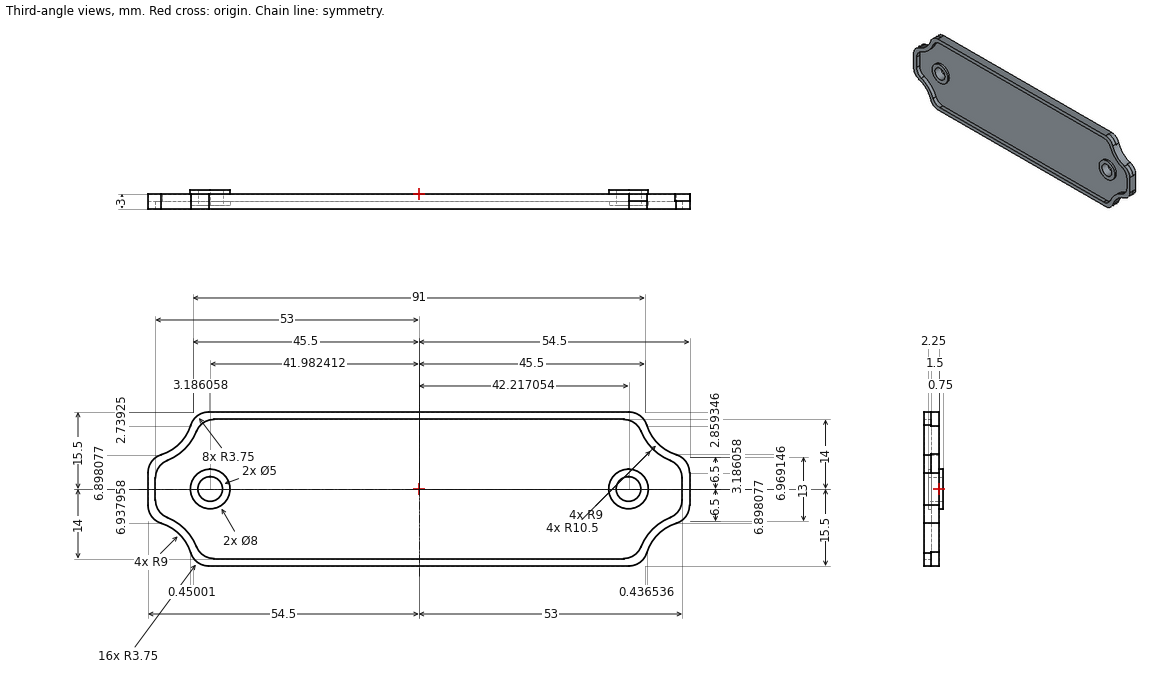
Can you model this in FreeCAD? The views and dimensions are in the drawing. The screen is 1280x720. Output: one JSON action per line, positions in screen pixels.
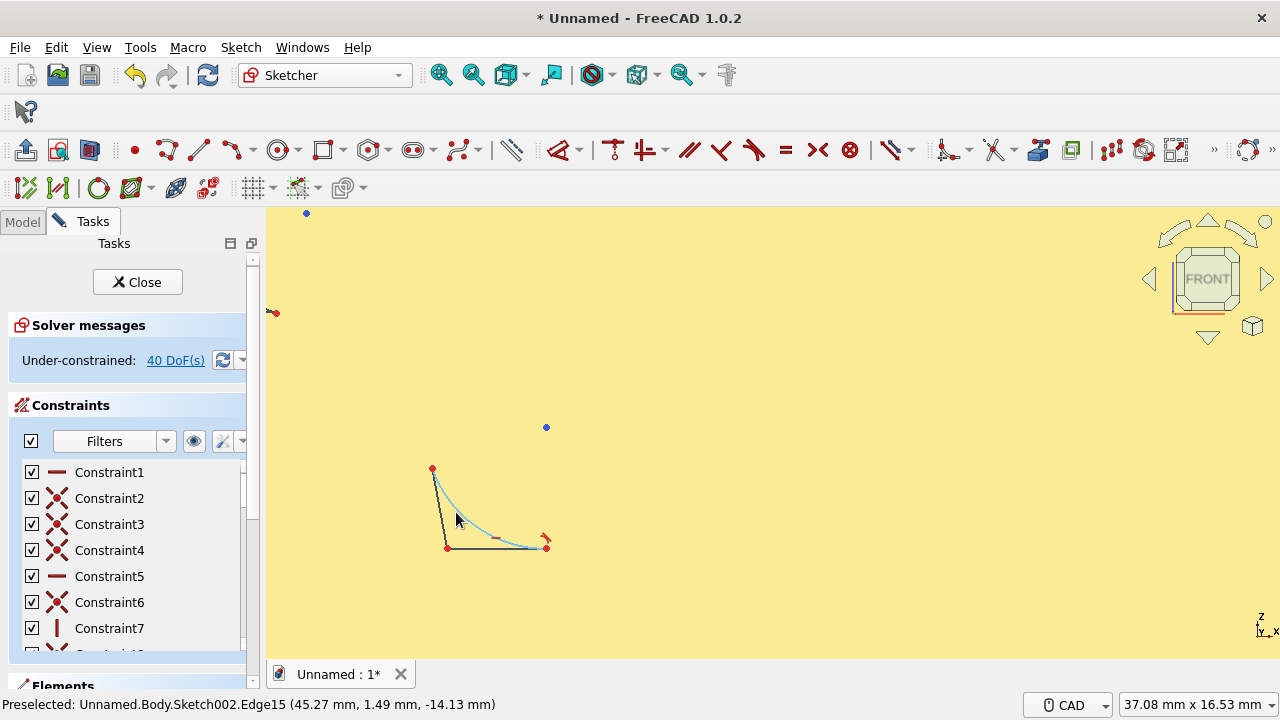
{"action": "left_click", "coordinate": [455, 507]}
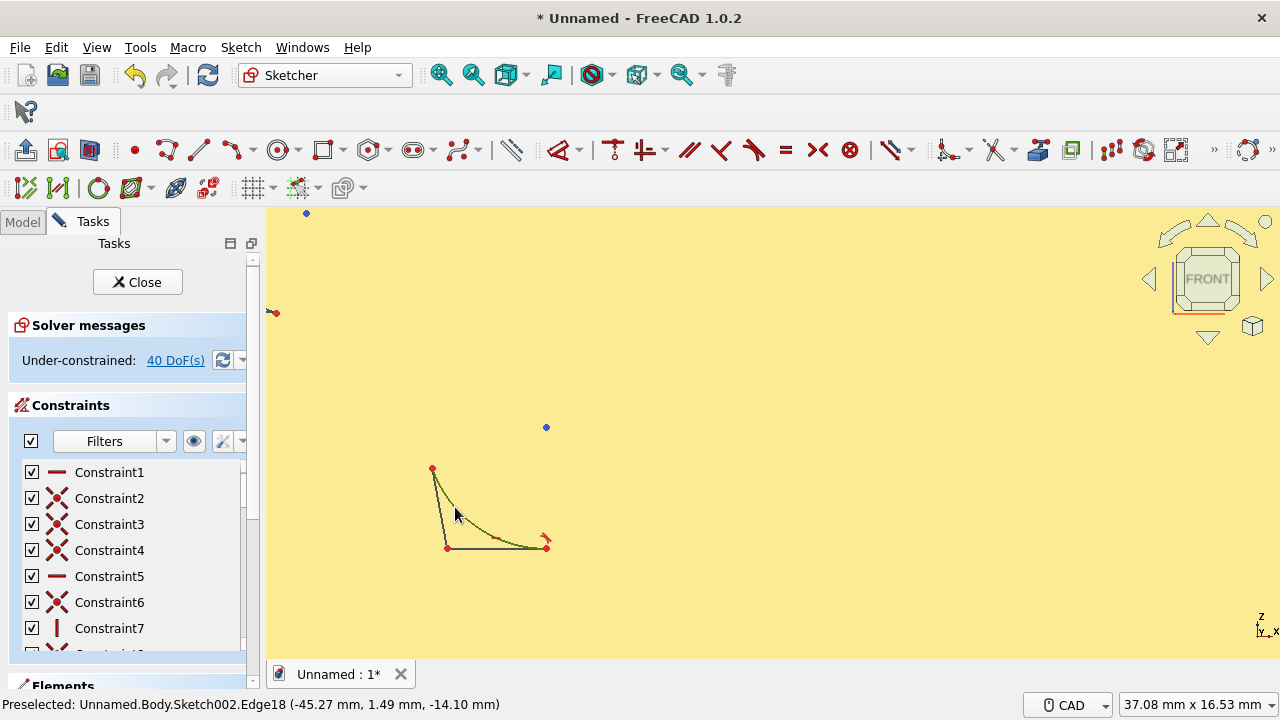
{"action": "scroll", "coordinate": [455, 512], "scroll_direction": "down", "scroll_amount": 8}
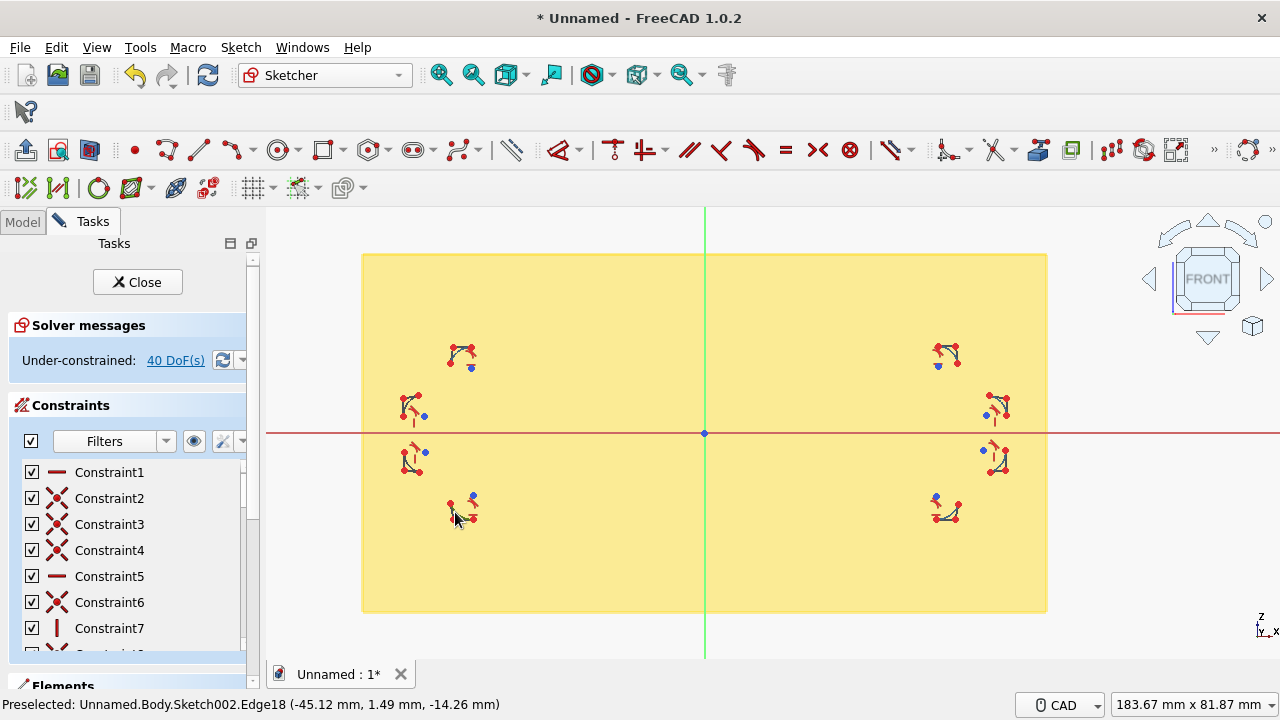
{"action": "scroll", "coordinate": [412, 469], "scroll_direction": "up", "scroll_amount": 9}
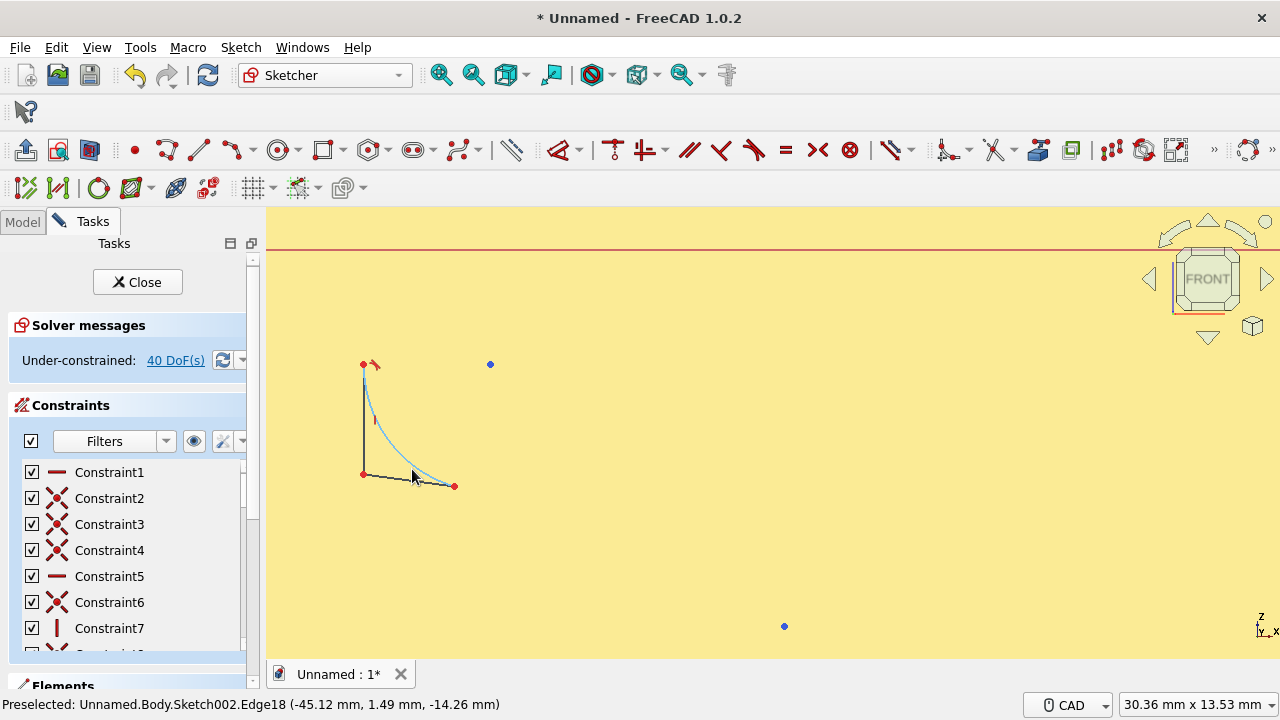
{"action": "left_click", "coordinate": [412, 464]}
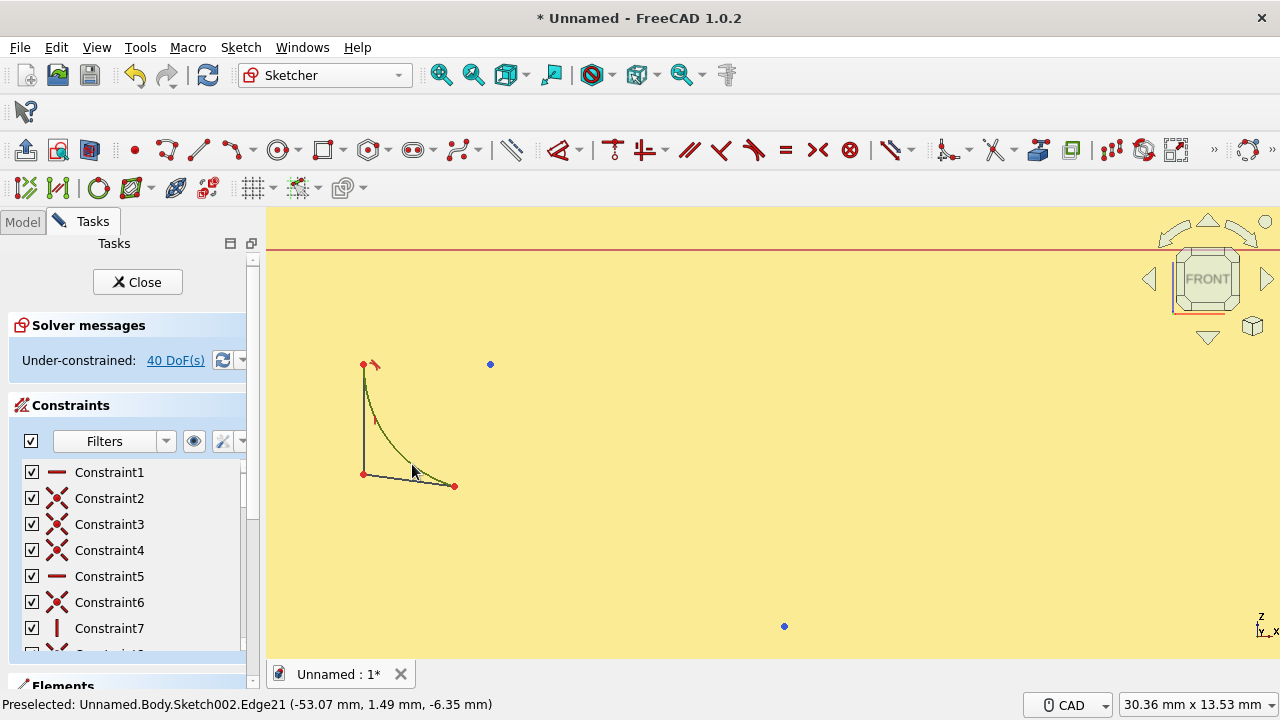
{"action": "scroll", "coordinate": [412, 469], "scroll_direction": "down", "scroll_amount": 9}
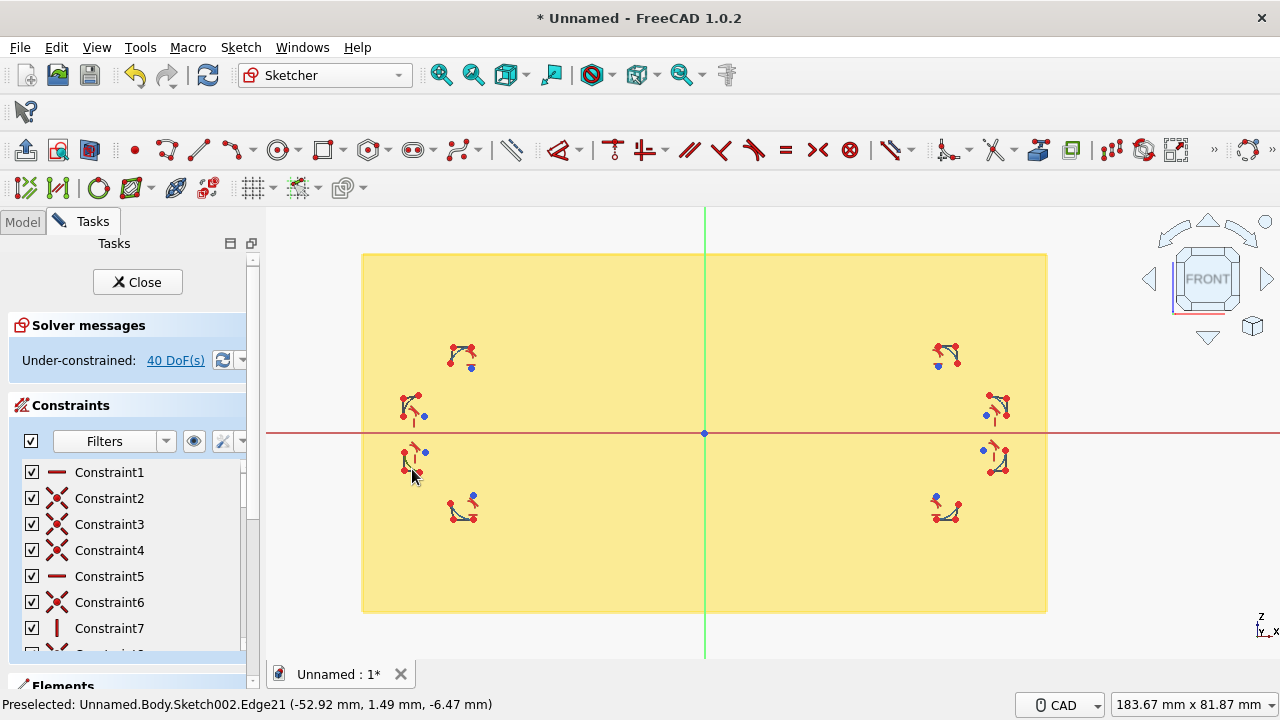
{"action": "scroll", "coordinate": [411, 400], "scroll_direction": "up", "scroll_amount": 9}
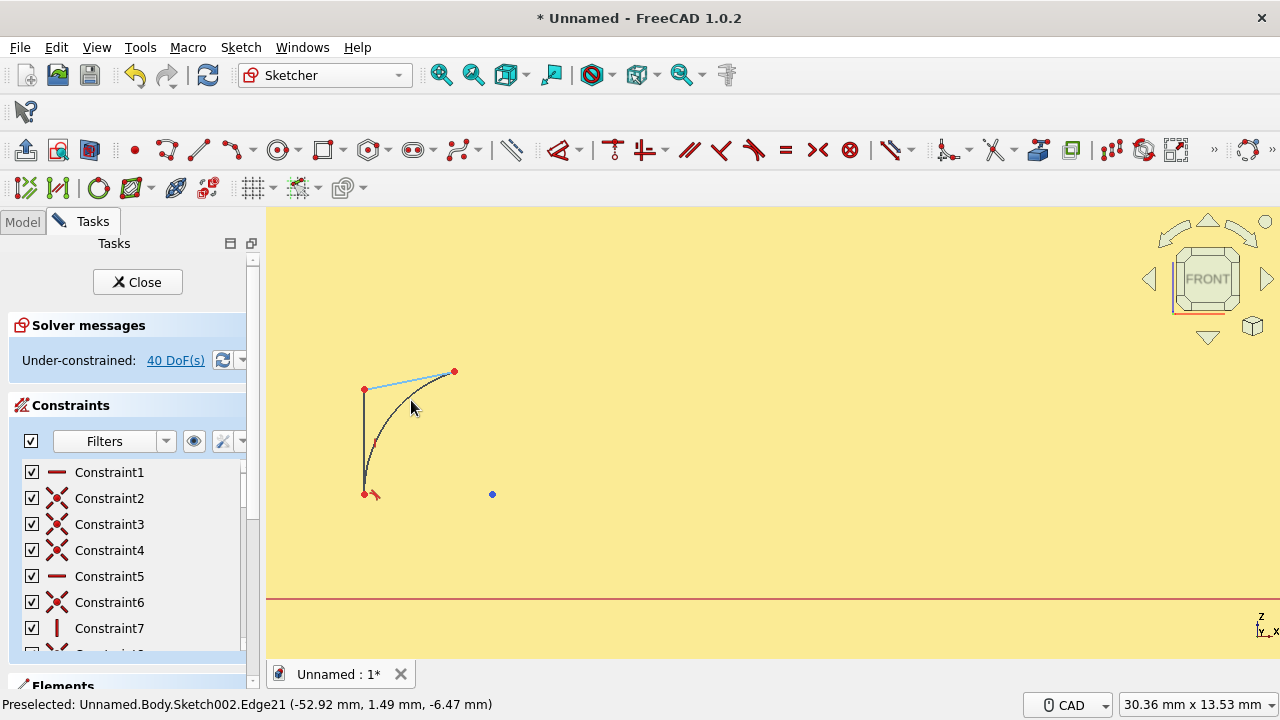
{"action": "left_click", "coordinate": [412, 395]}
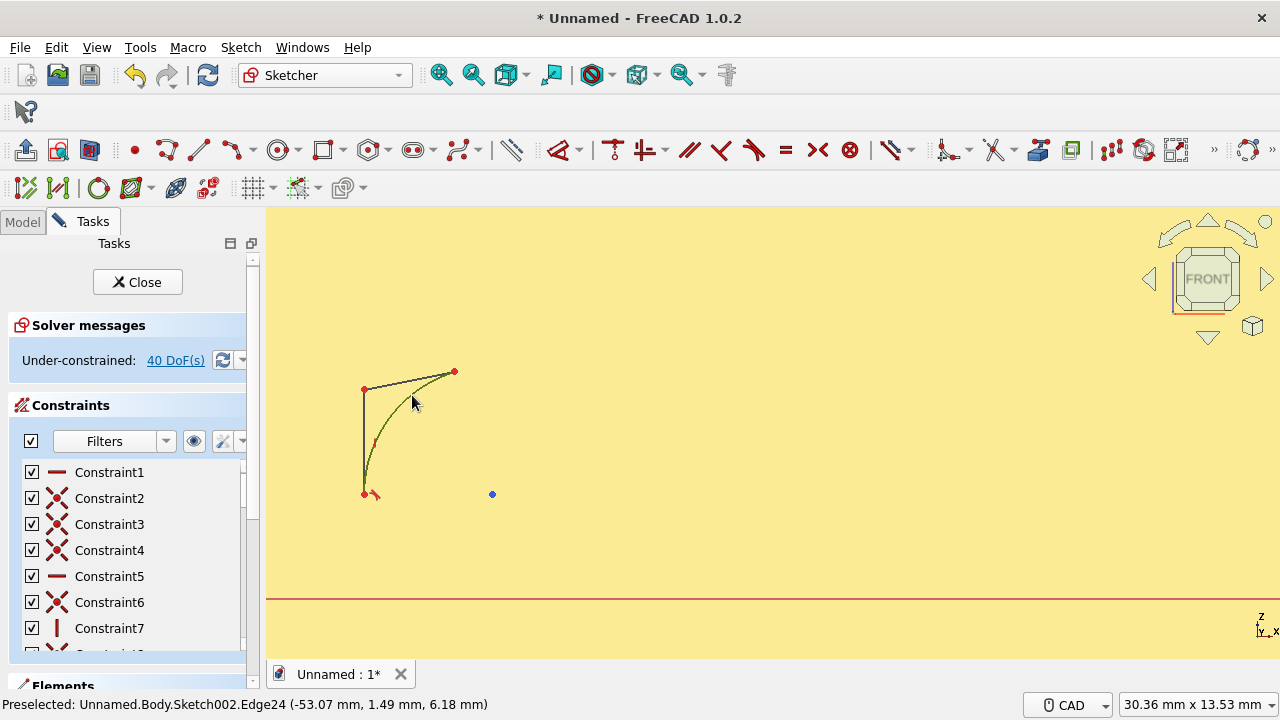
{"action": "left_click", "coordinate": [786, 150]}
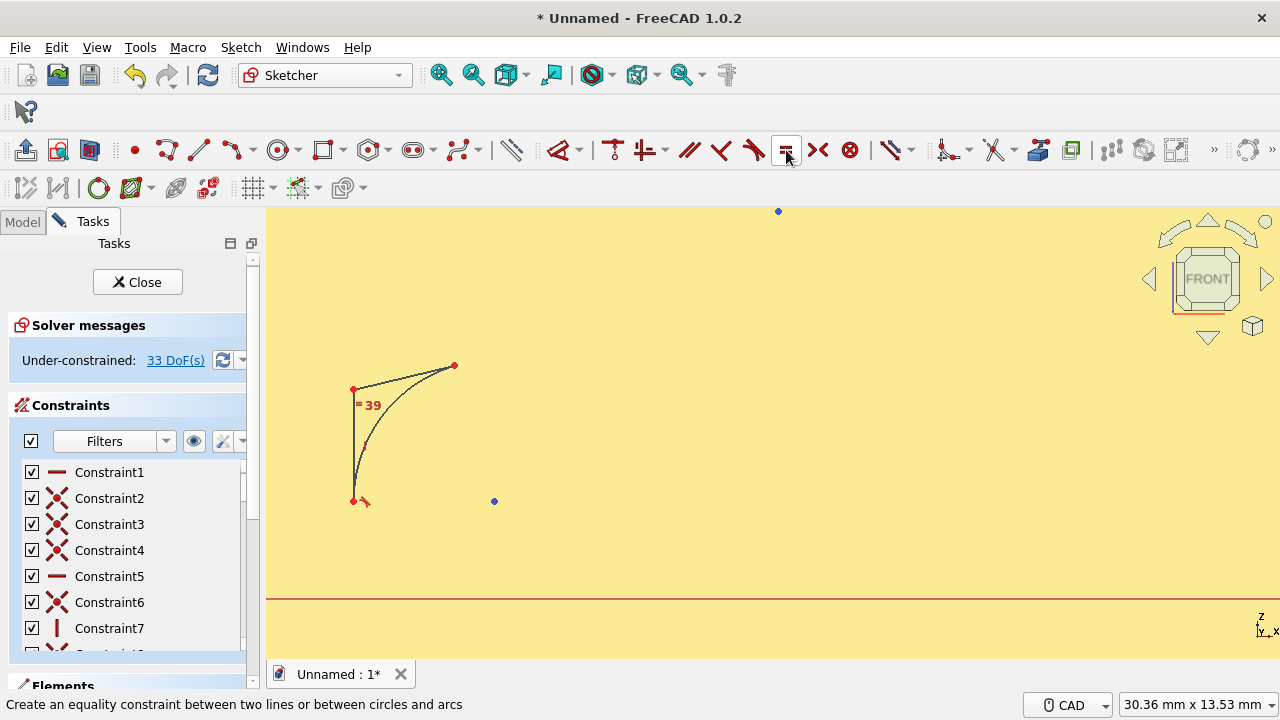
{"action": "scroll", "coordinate": [411, 400], "scroll_direction": "down", "scroll_amount": 9}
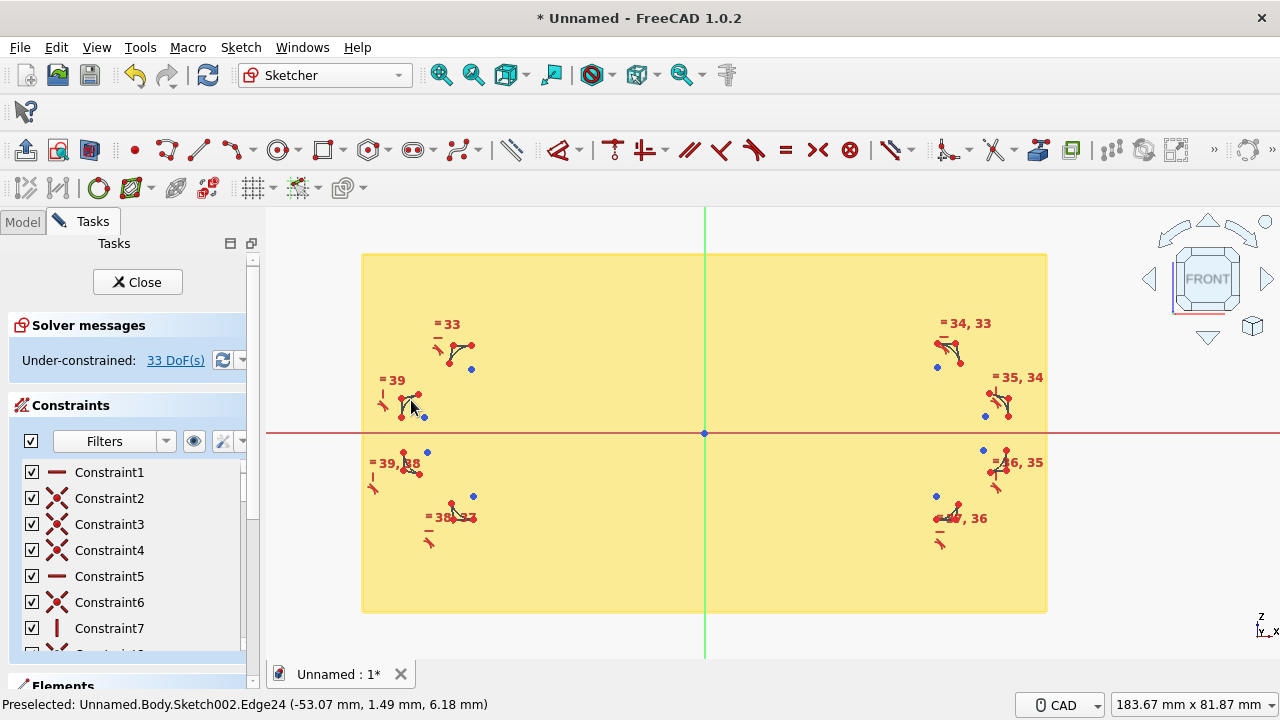
{"action": "left_click", "coordinate": [472, 369]}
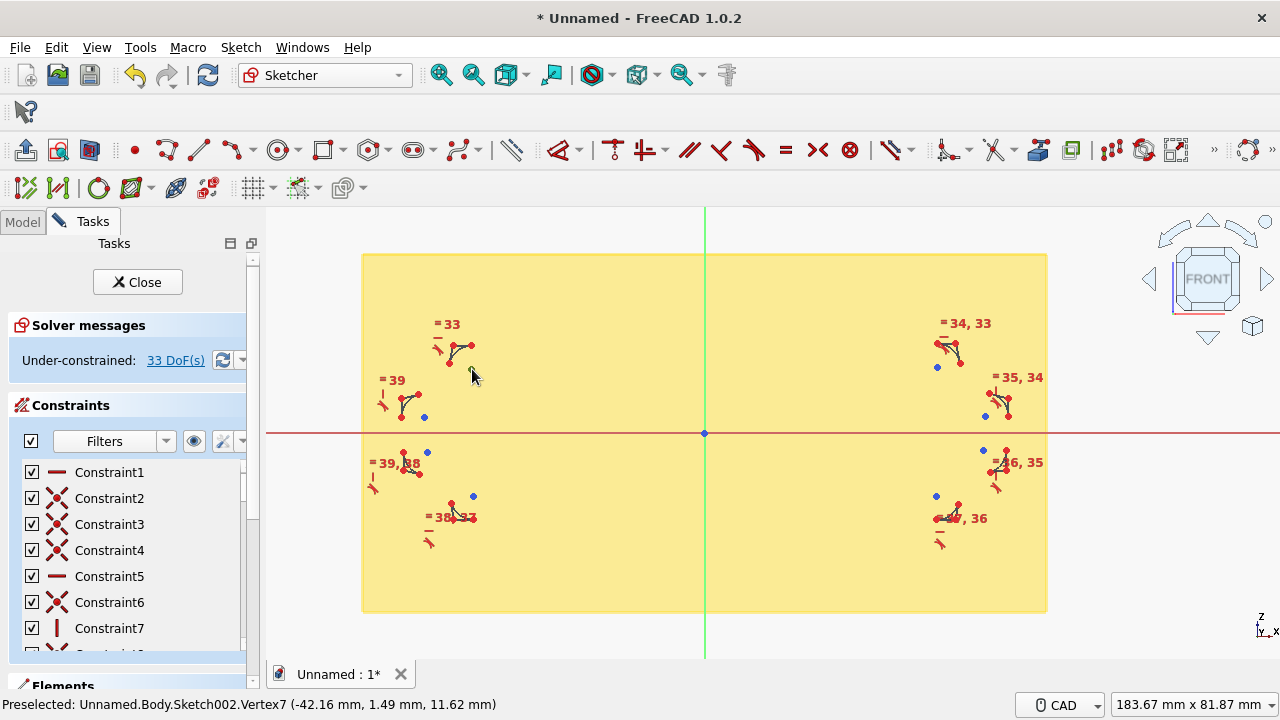
{"action": "left_click", "coordinate": [937, 367]}